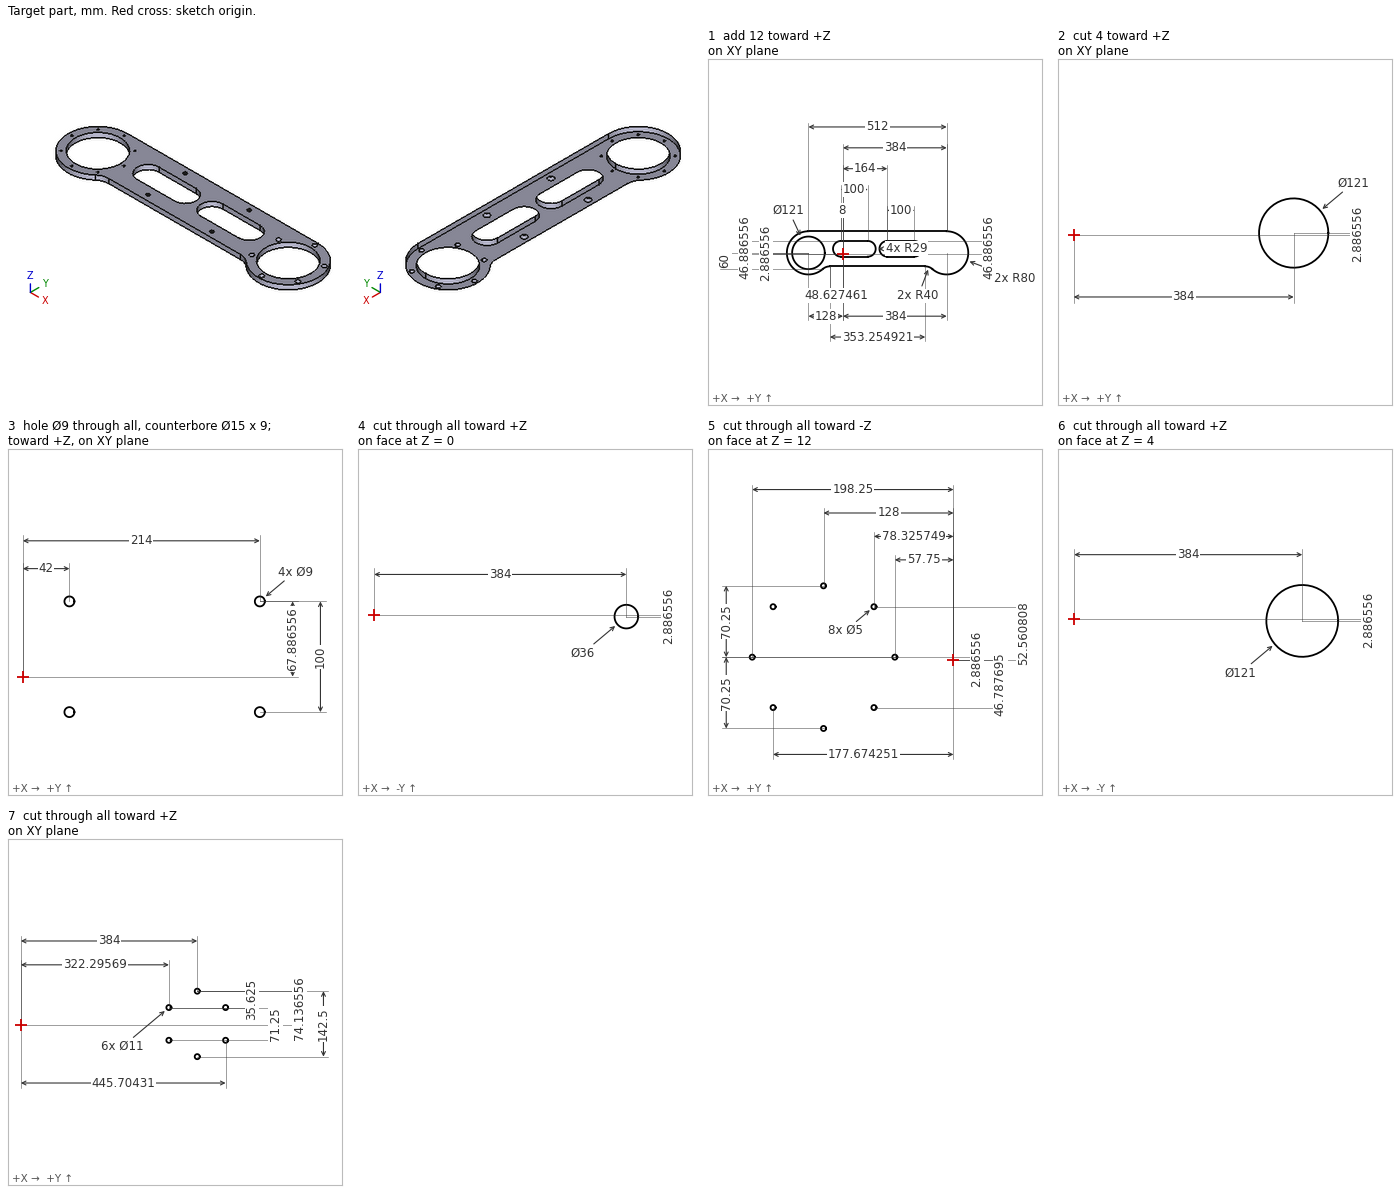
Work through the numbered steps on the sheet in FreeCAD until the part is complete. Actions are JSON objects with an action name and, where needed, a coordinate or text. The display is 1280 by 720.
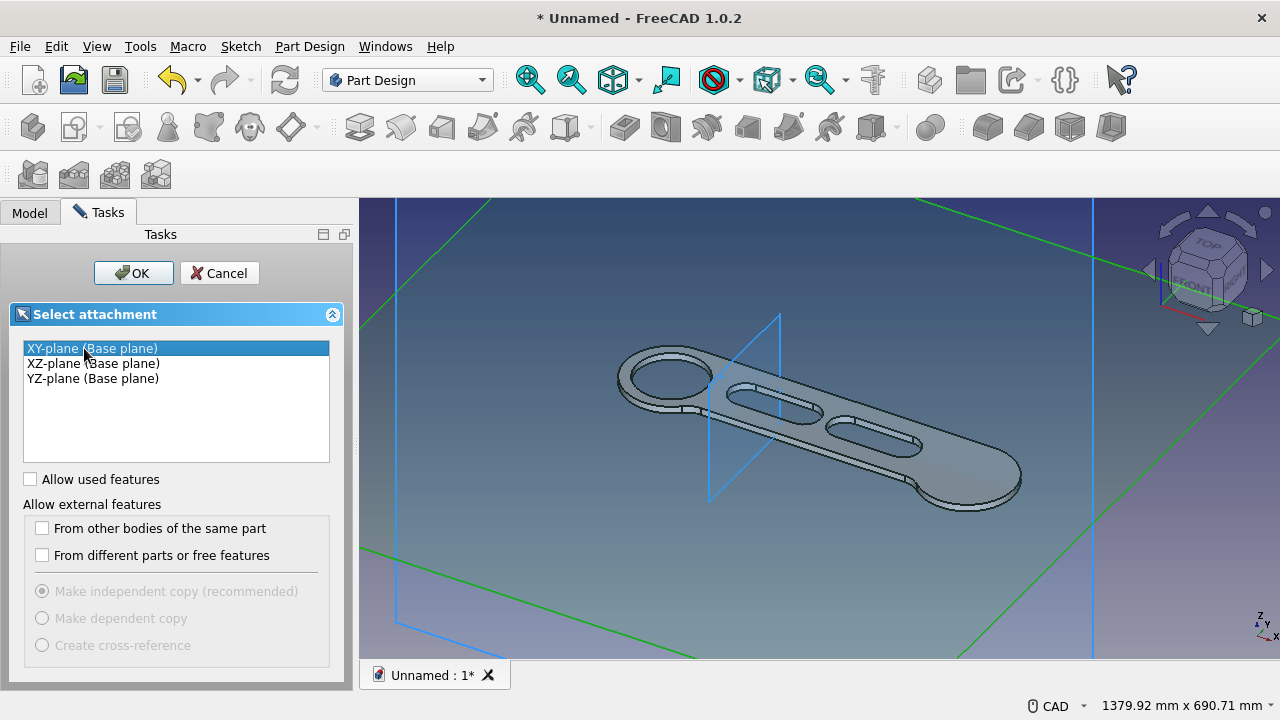
{"action": "left_click", "coordinate": [134, 273]}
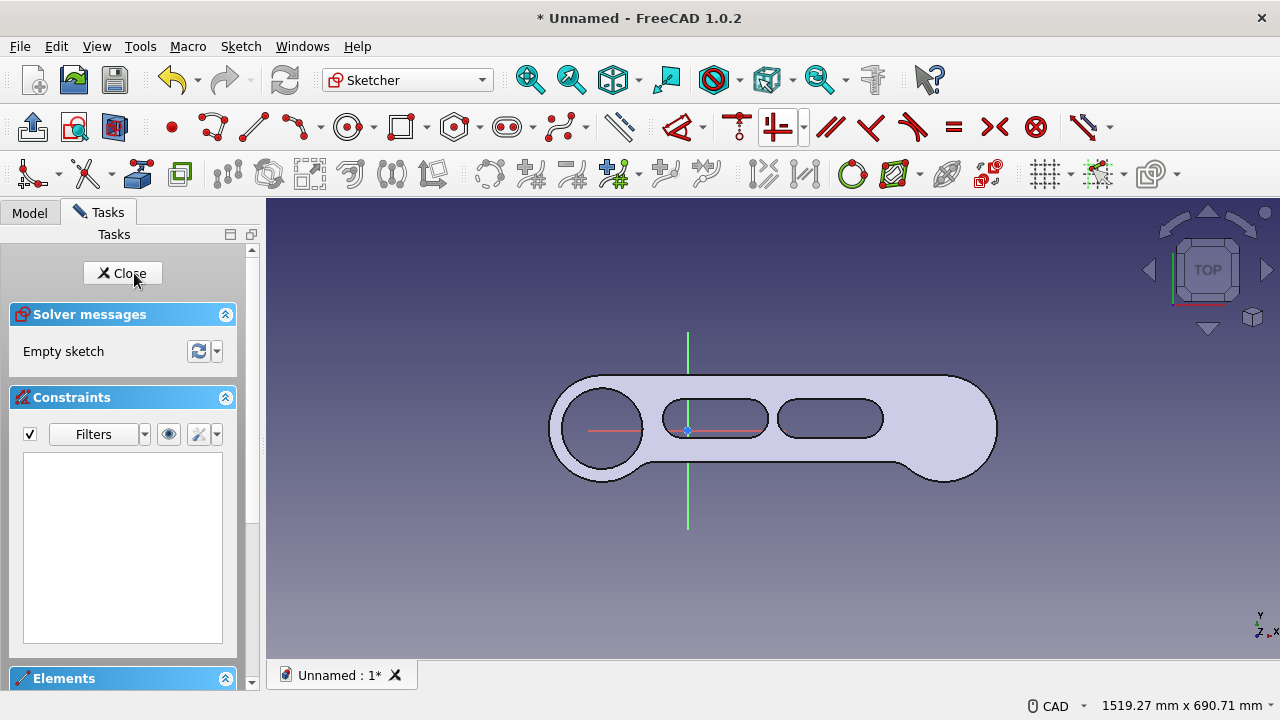
{"action": "left_click", "coordinate": [115, 128]}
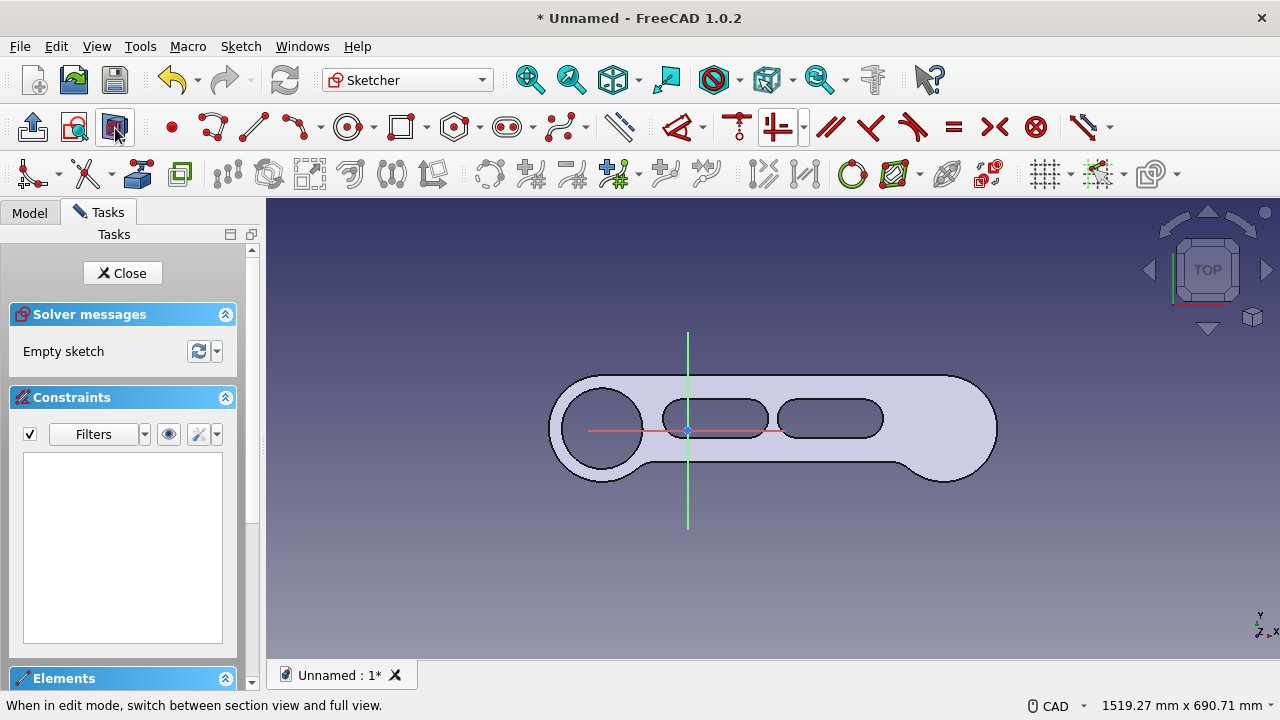
{"action": "scroll", "coordinate": [1047, 429], "scroll_direction": "up", "scroll_amount": 6}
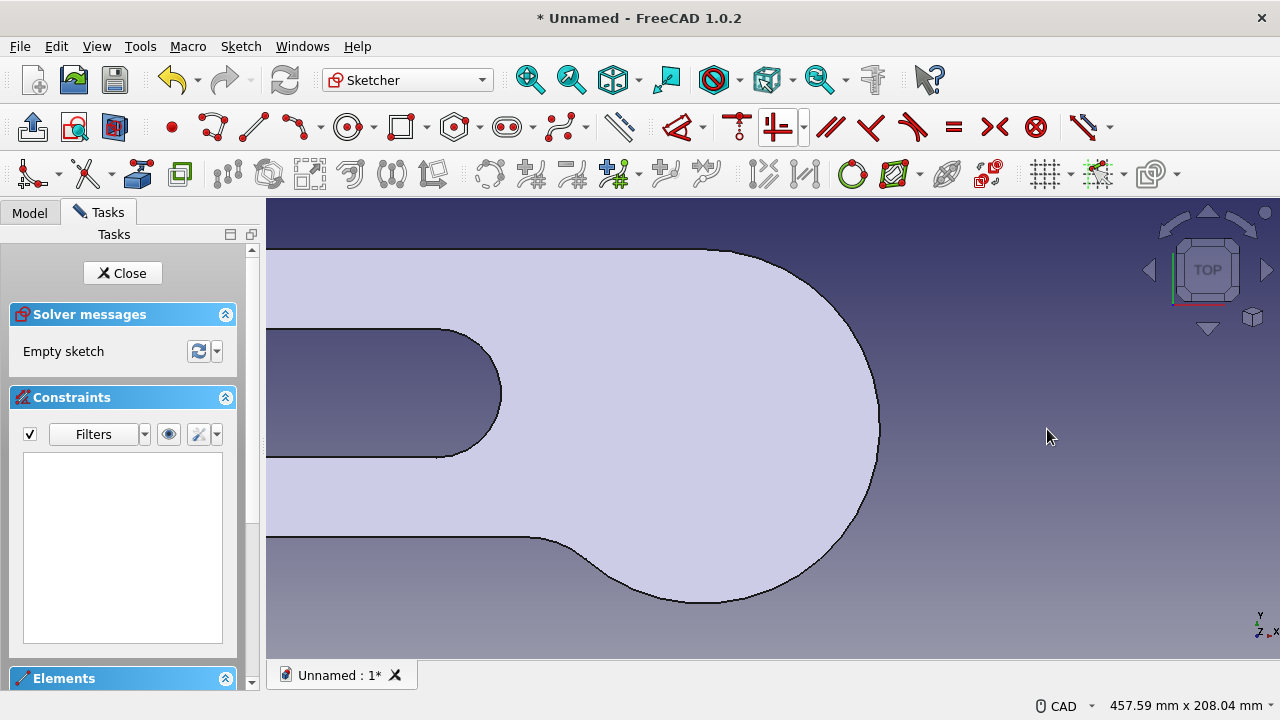
{"action": "left_click", "coordinate": [348, 128]}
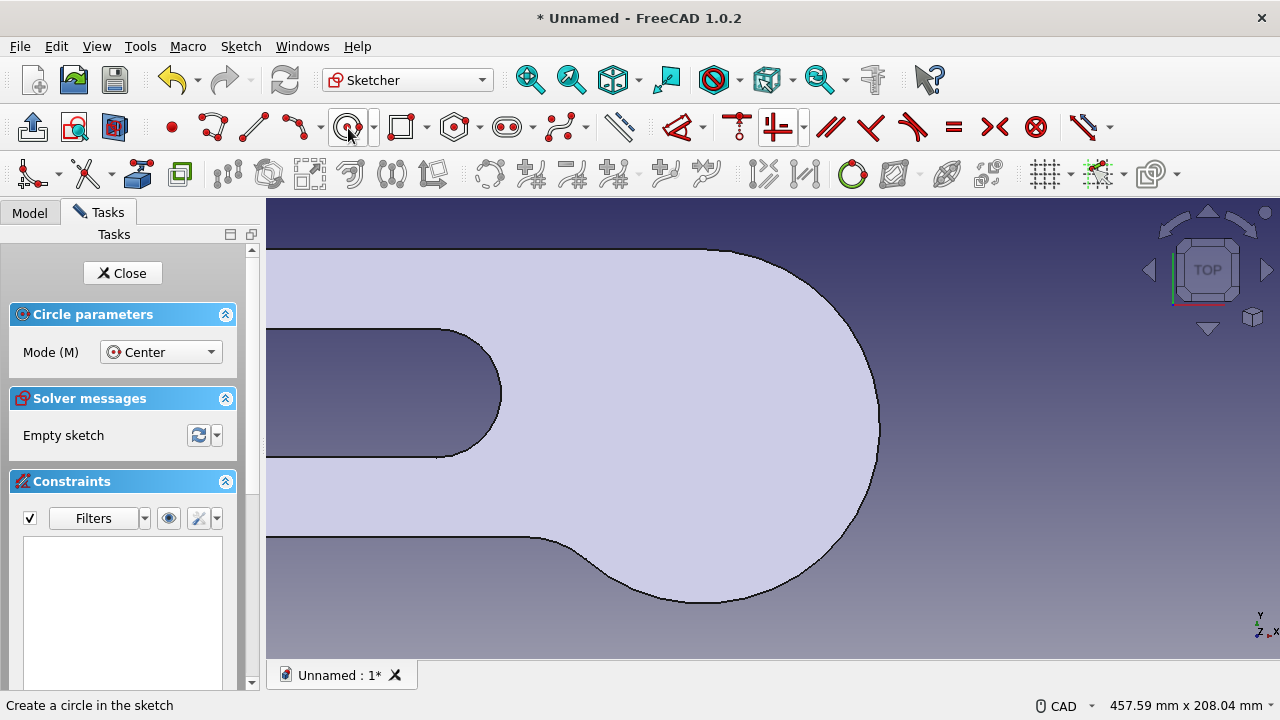
{"action": "scroll", "coordinate": [703, 426], "scroll_direction": "up", "scroll_amount": 5}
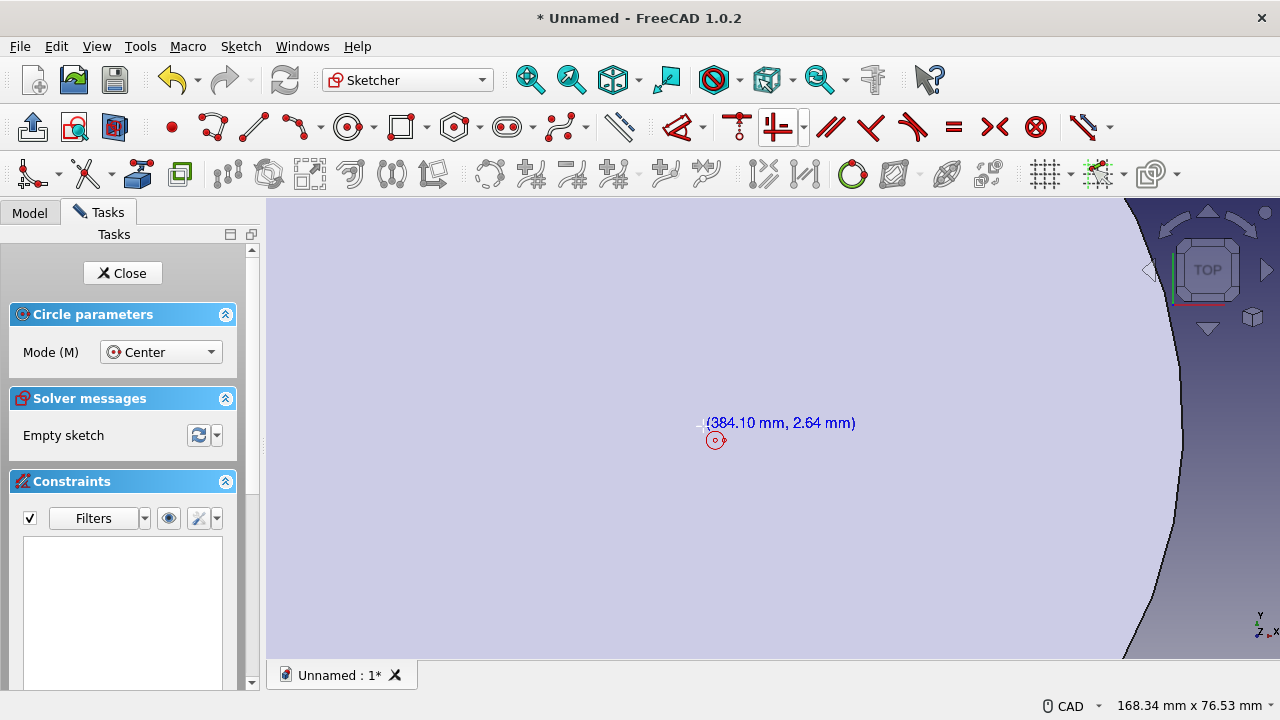
{"action": "left_click", "coordinate": [702, 426]}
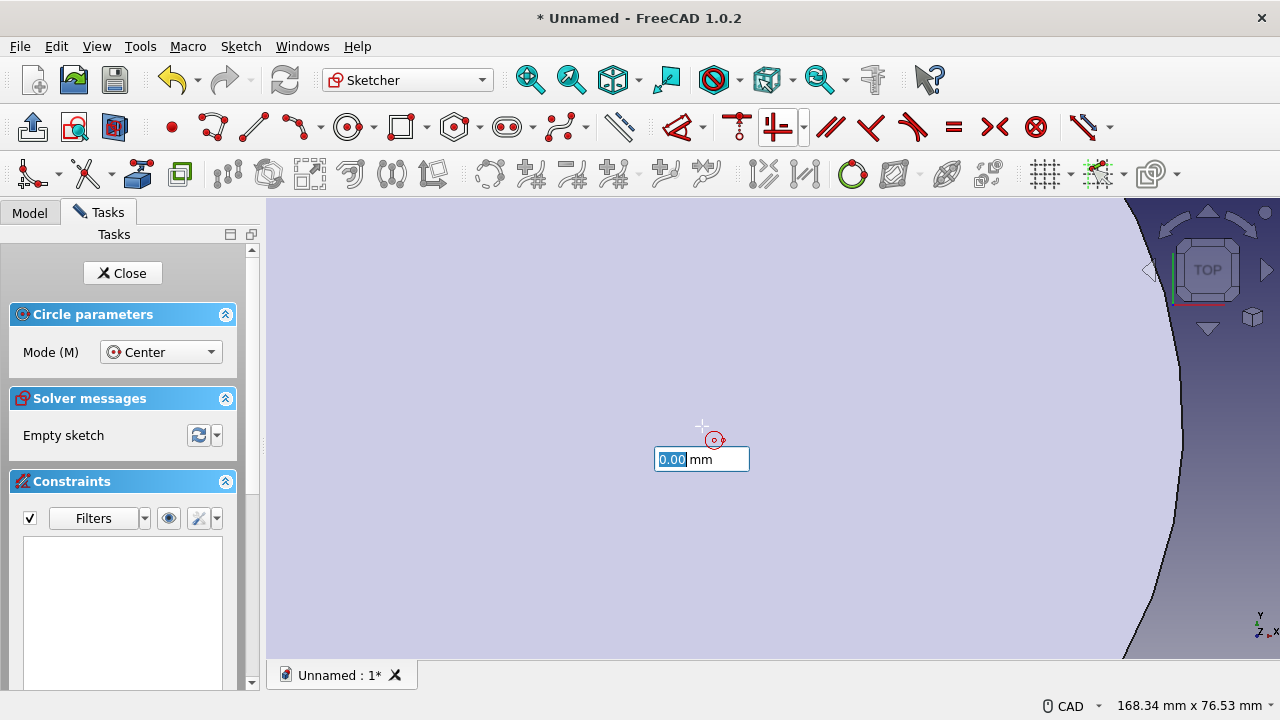
{"action": "scroll", "coordinate": [706, 430], "scroll_direction": "down", "scroll_amount": 5}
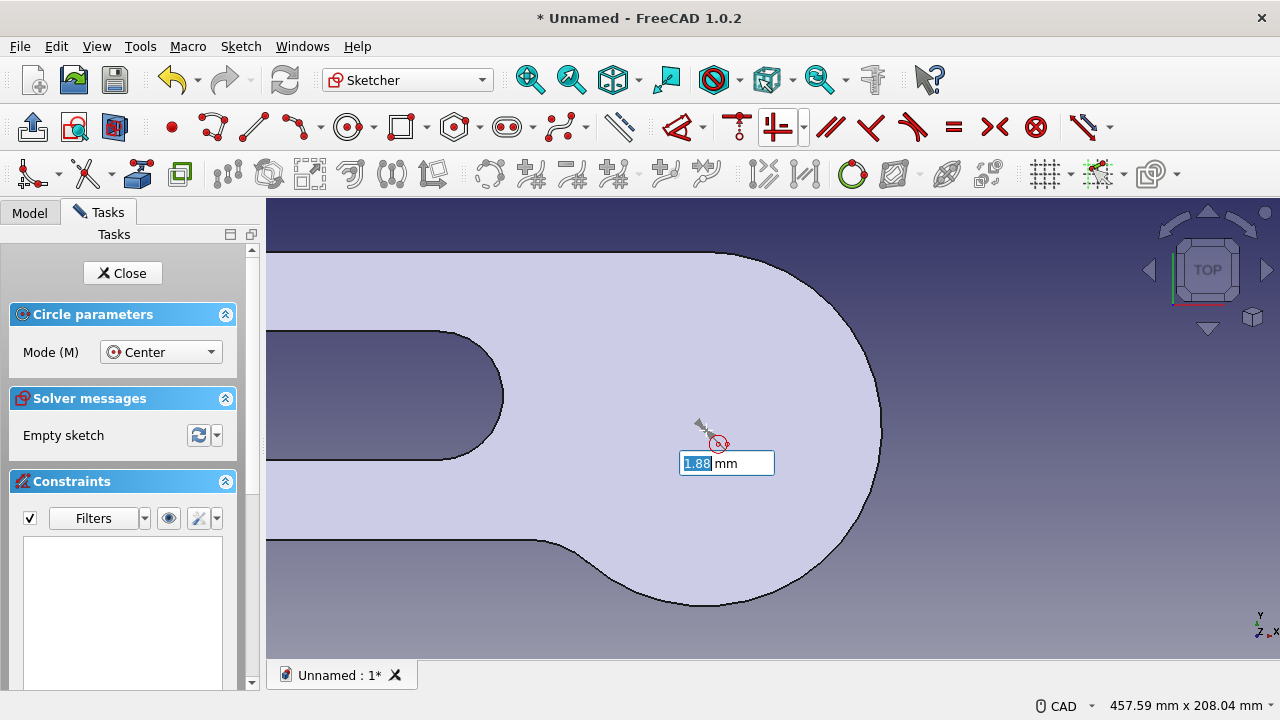
{"action": "left_click", "coordinate": [799, 334]}
{"action": "key", "text": "Escape"}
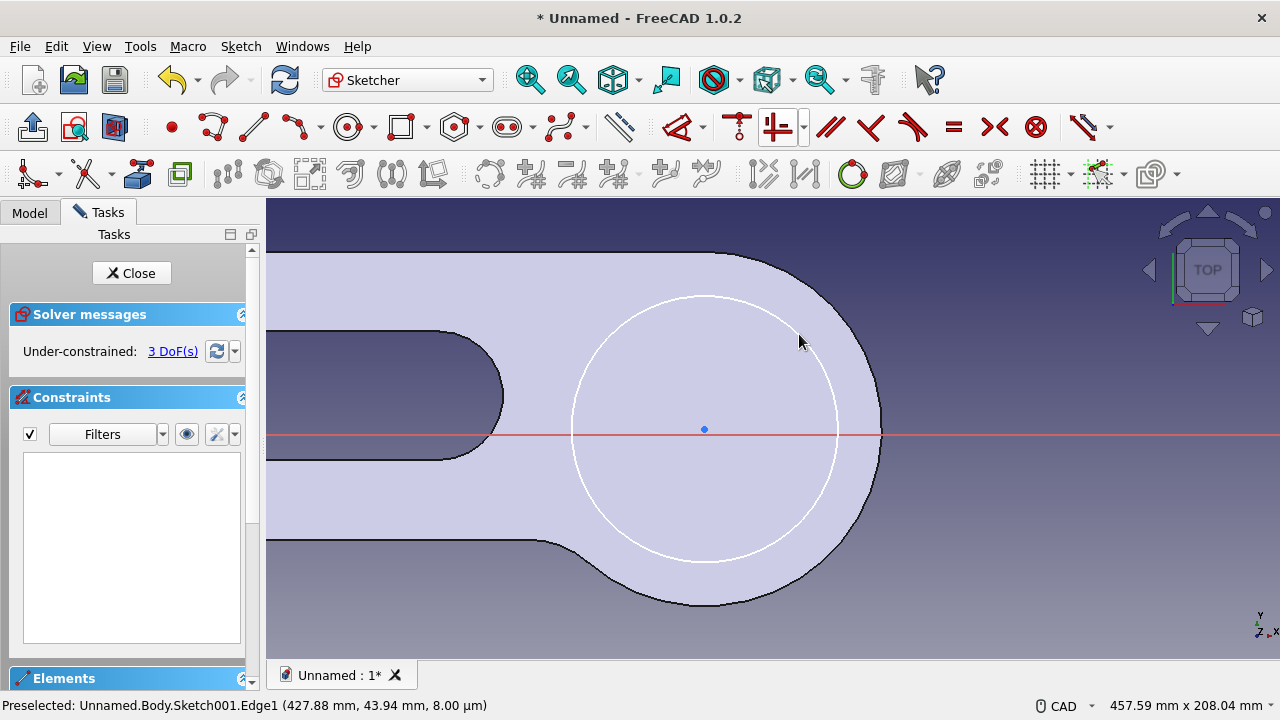
{"action": "left_click", "coordinate": [676, 128]}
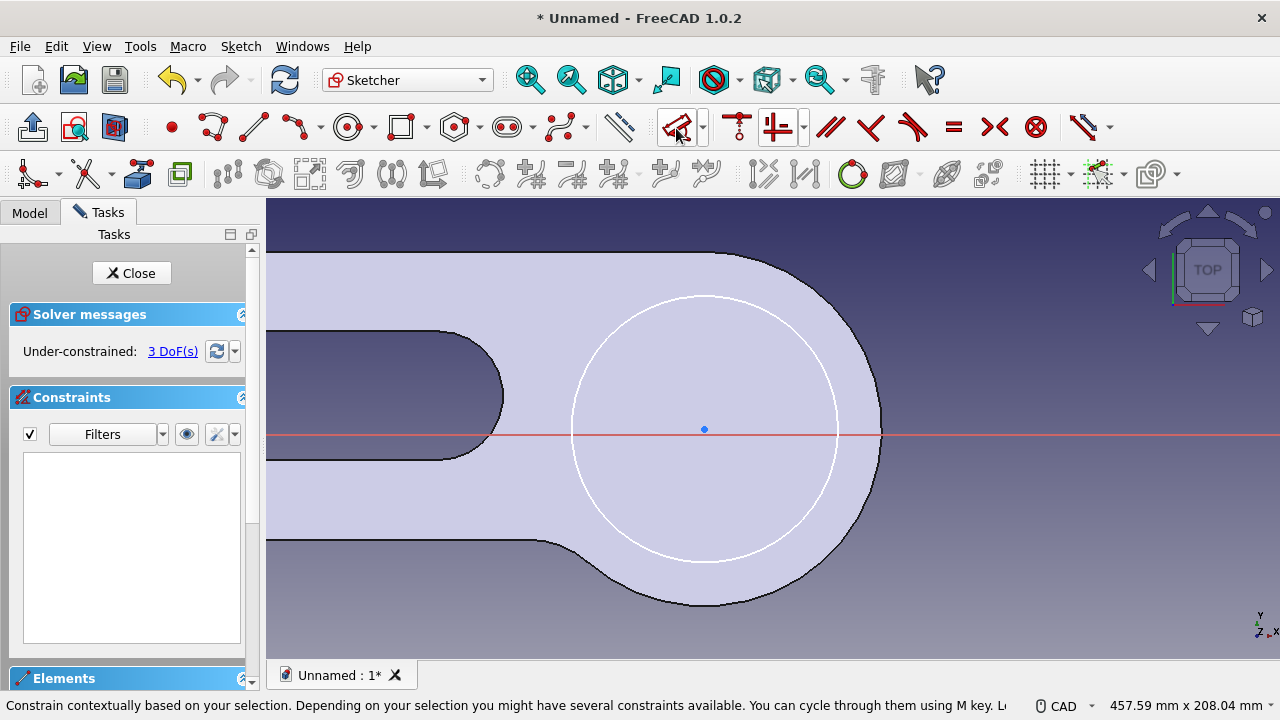
{"action": "left_click", "coordinate": [799, 335]}
{"action": "left_click", "coordinate": [822, 312]}